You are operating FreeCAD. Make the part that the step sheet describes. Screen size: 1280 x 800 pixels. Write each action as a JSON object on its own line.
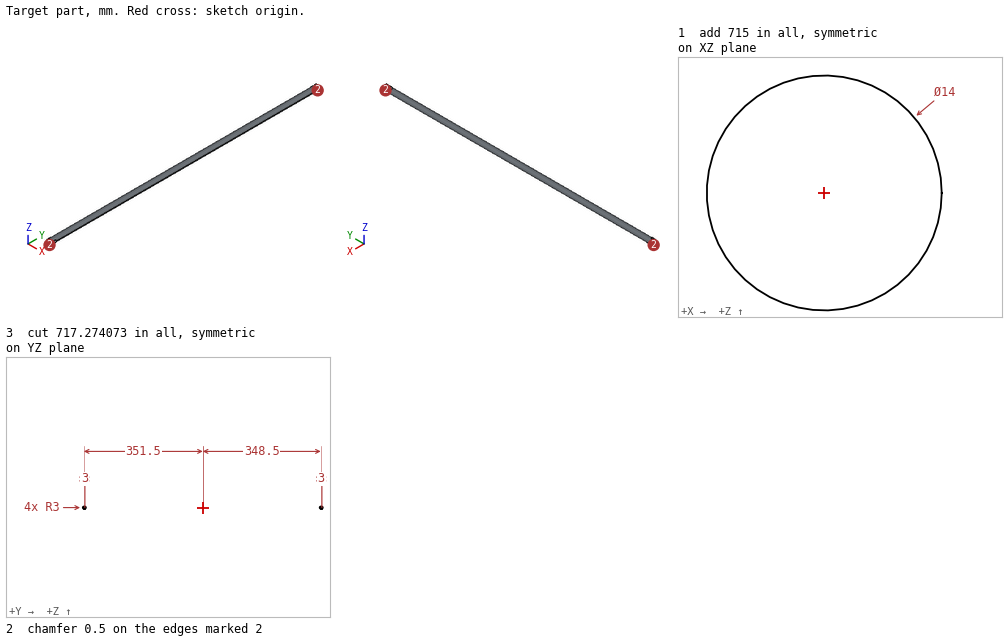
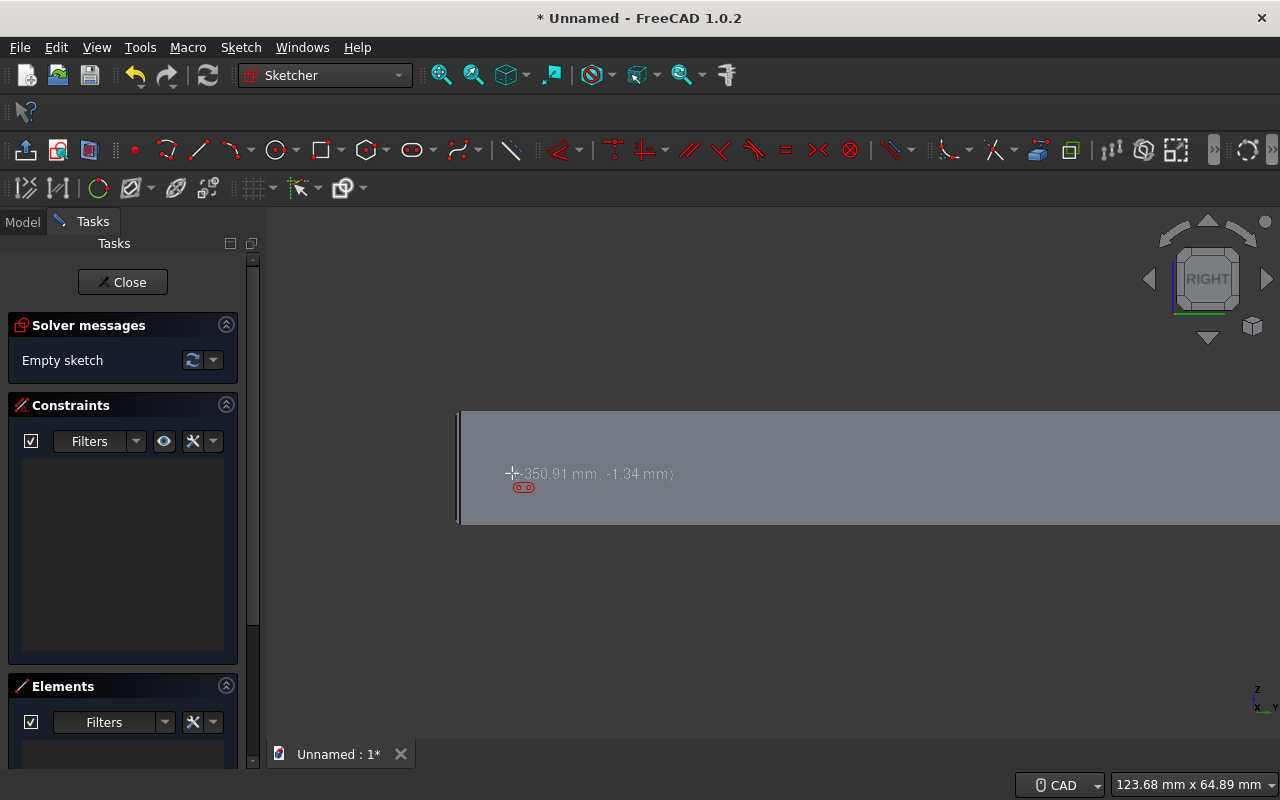
{"action": "scroll", "coordinate": [437, 474], "scroll_direction": "down", "scroll_amount": 12}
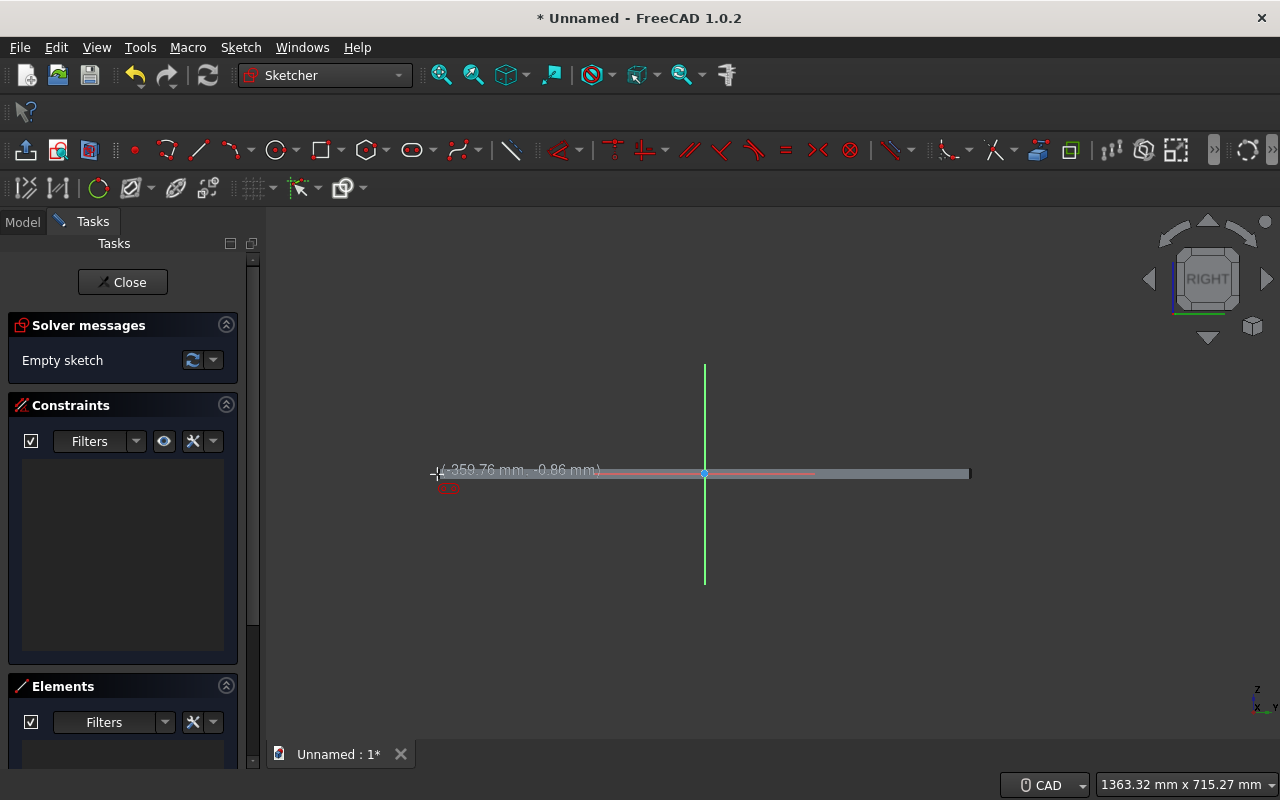
{"action": "left_click", "coordinate": [443, 474]}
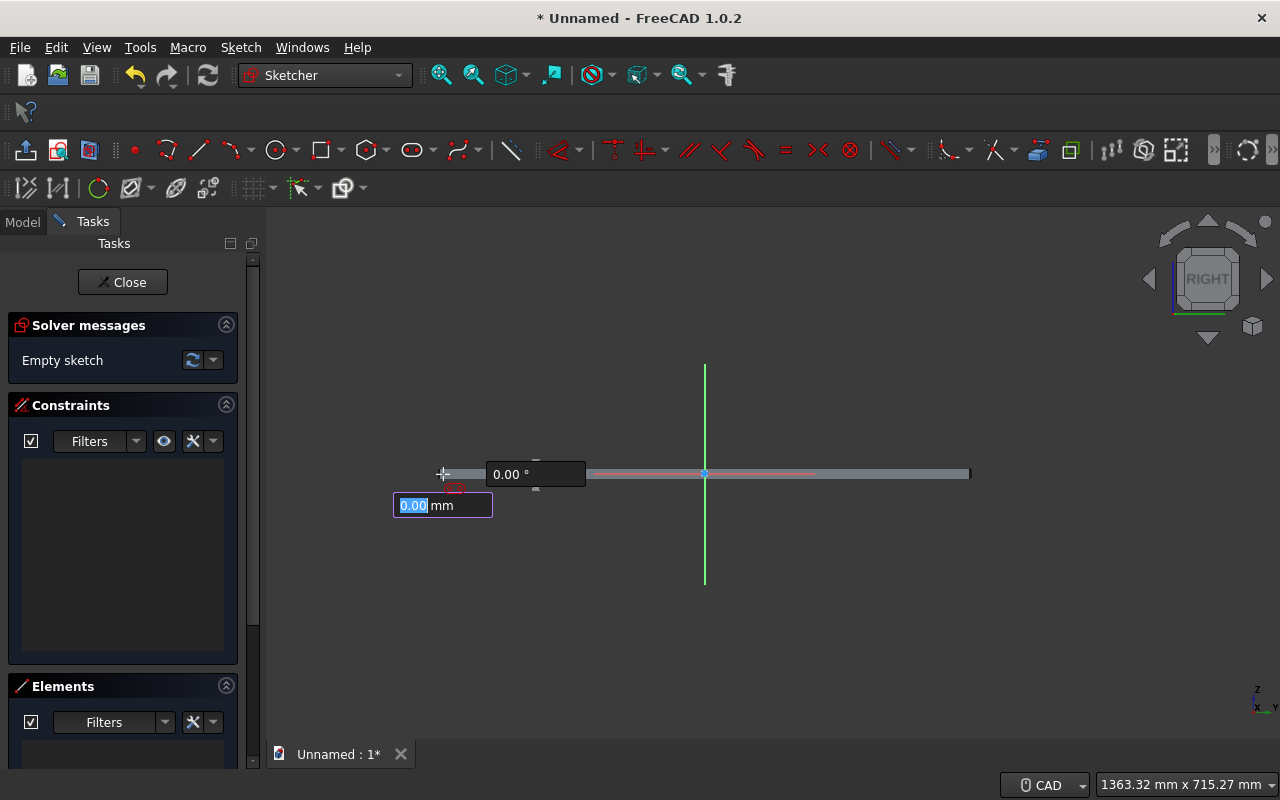
{"action": "scroll", "coordinate": [446, 474], "scroll_direction": "up", "scroll_amount": 10}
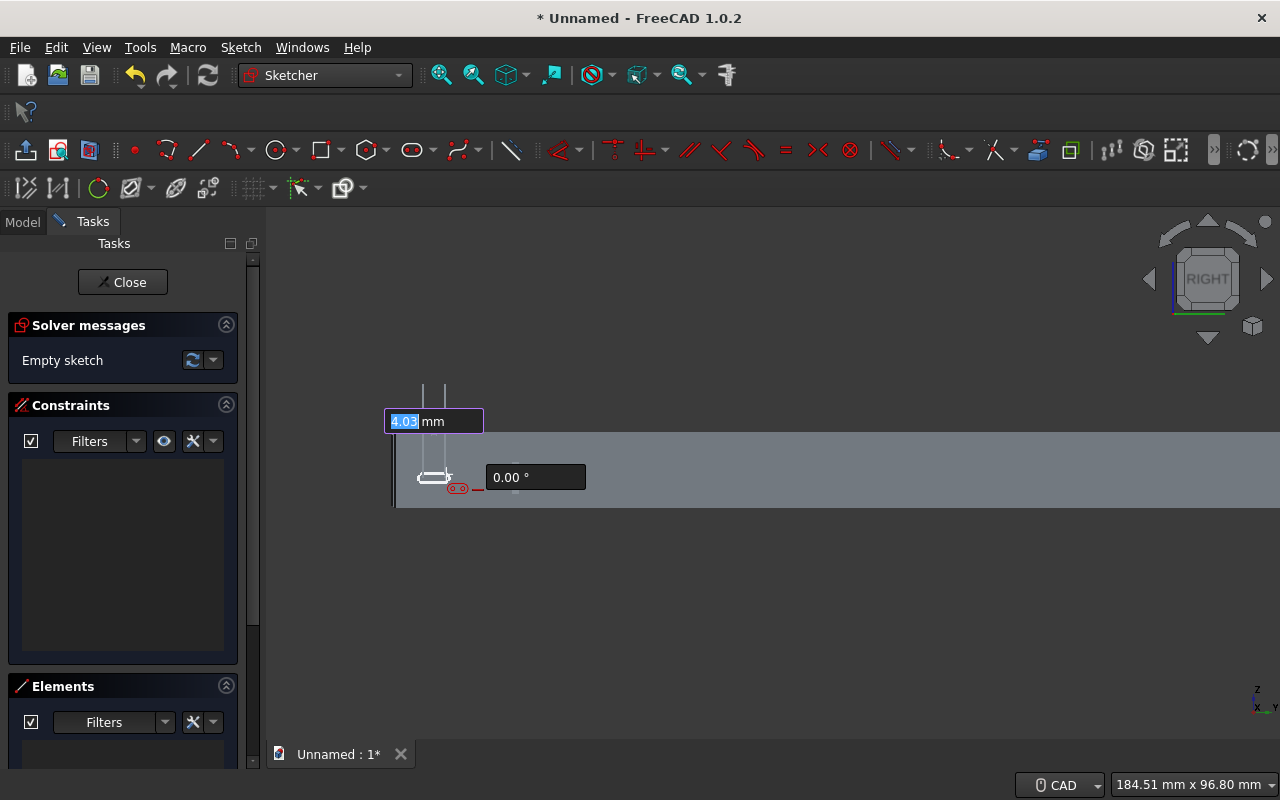
{"action": "left_click", "coordinate": [441, 461]}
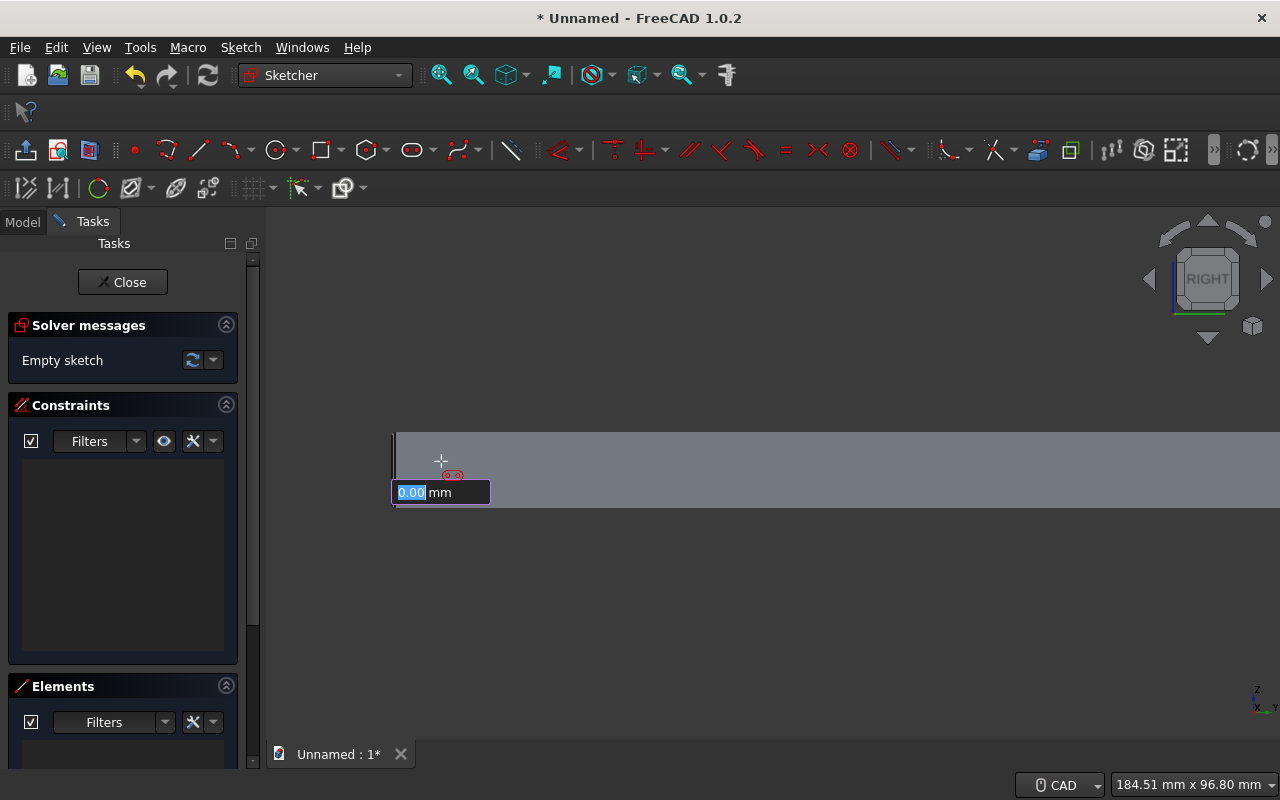
{"action": "left_click", "coordinate": [433, 454]}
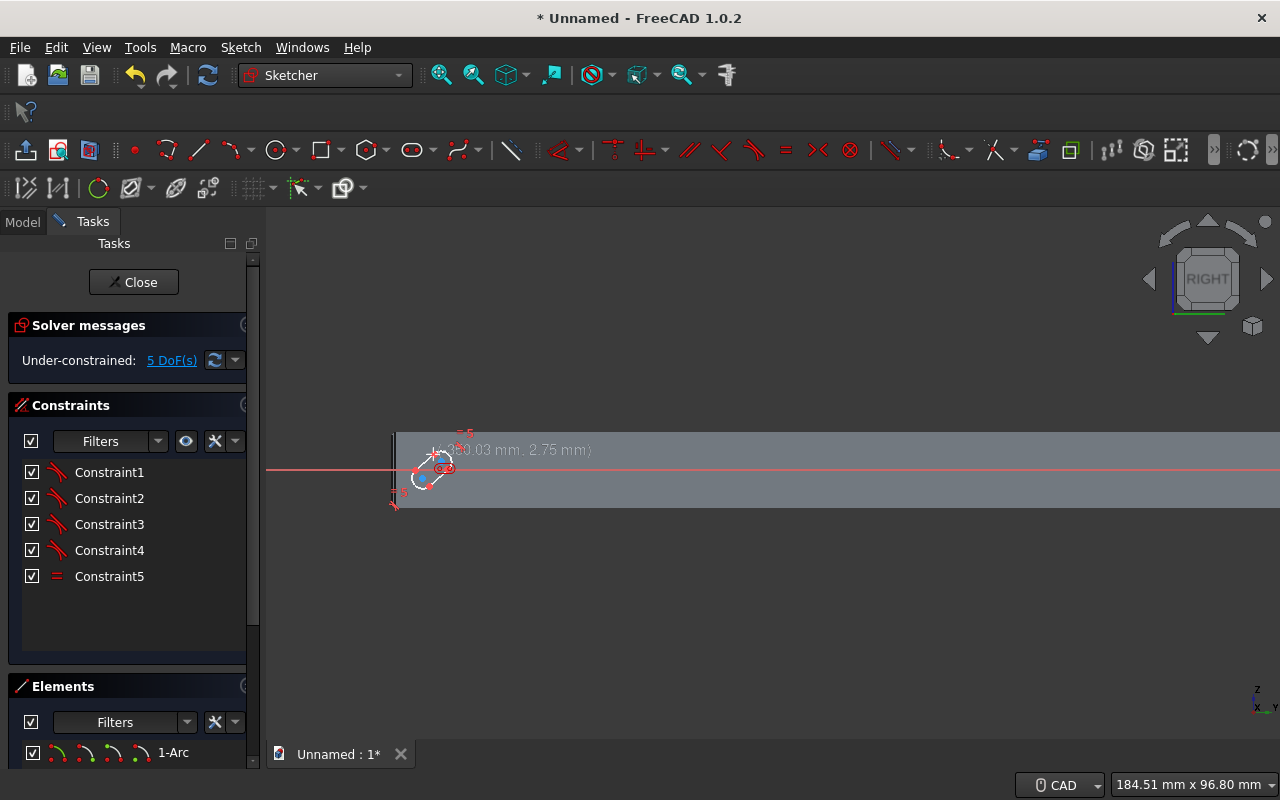
{"action": "scroll", "coordinate": [446, 473], "scroll_direction": "down", "scroll_amount": 10}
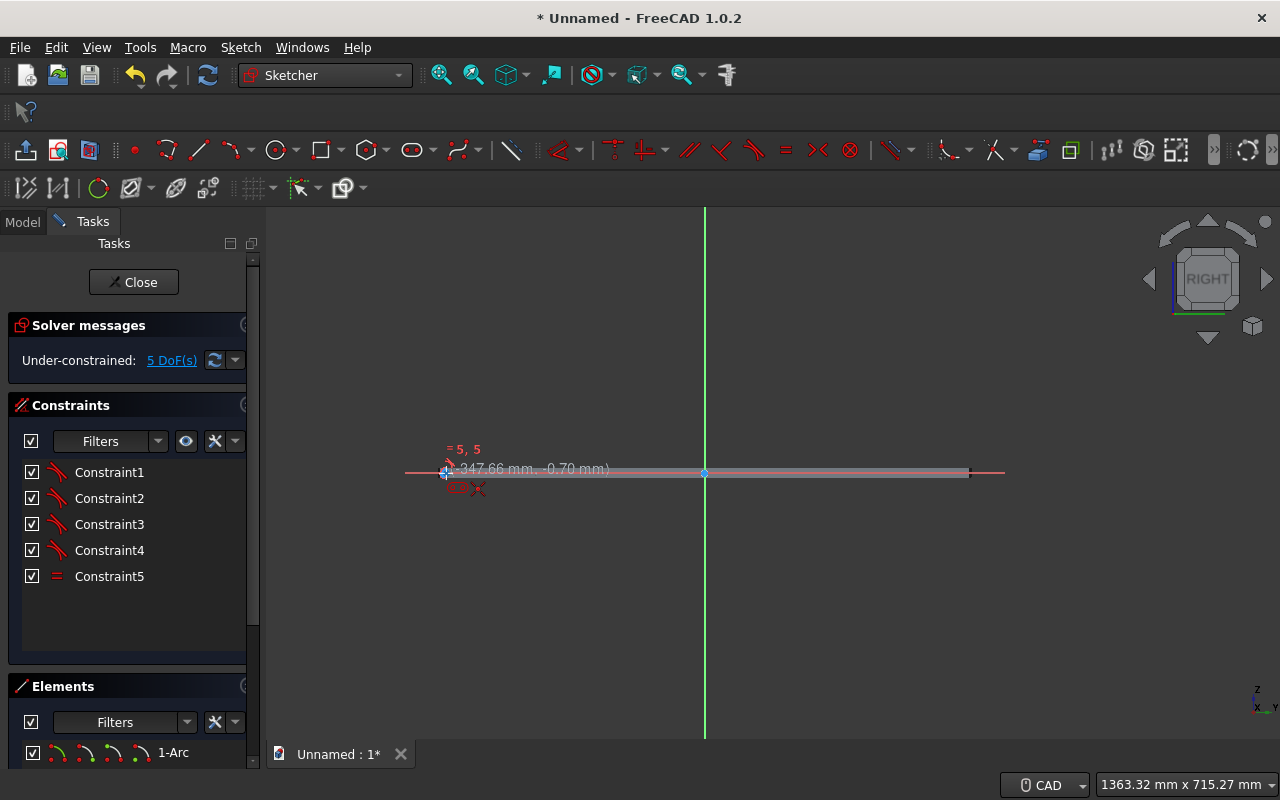
{"action": "scroll", "coordinate": [964, 473], "scroll_direction": "up", "scroll_amount": 12}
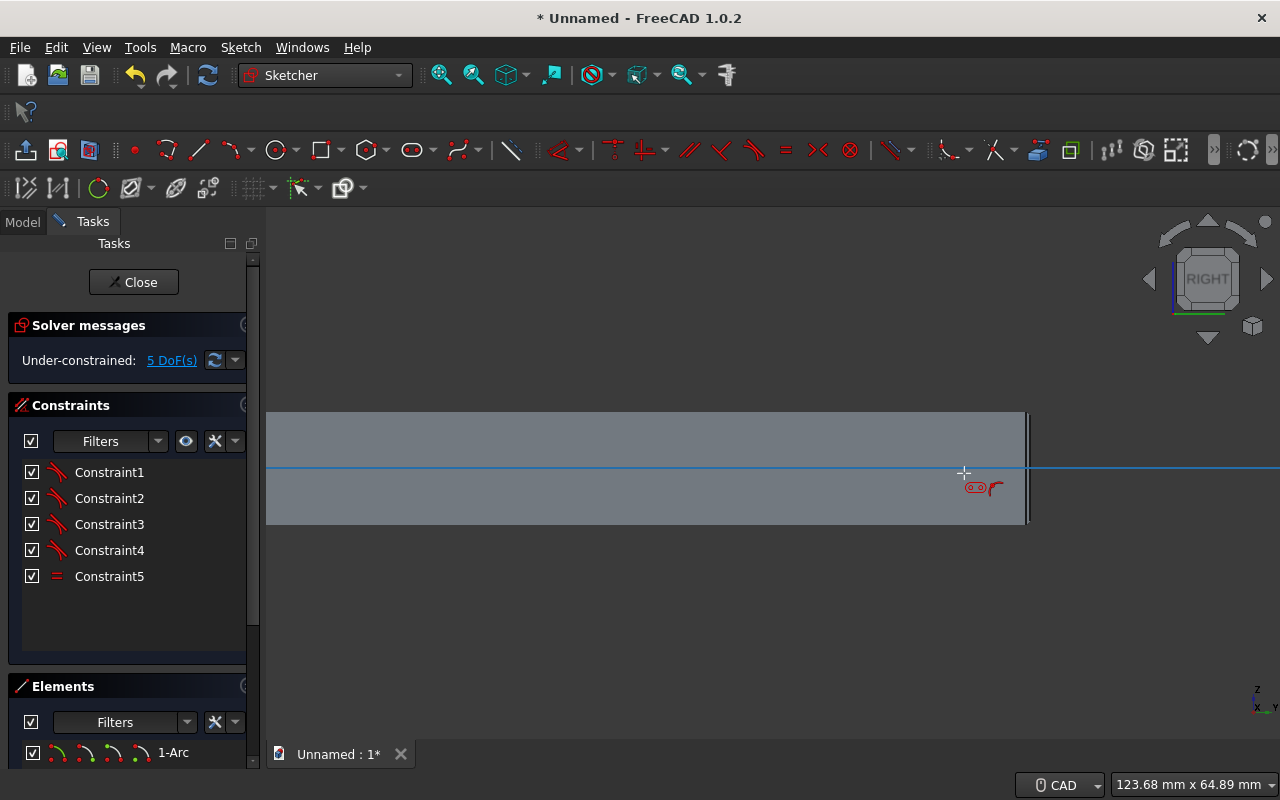
{"action": "scroll", "coordinate": [964, 473], "scroll_direction": "down", "scroll_amount": 12}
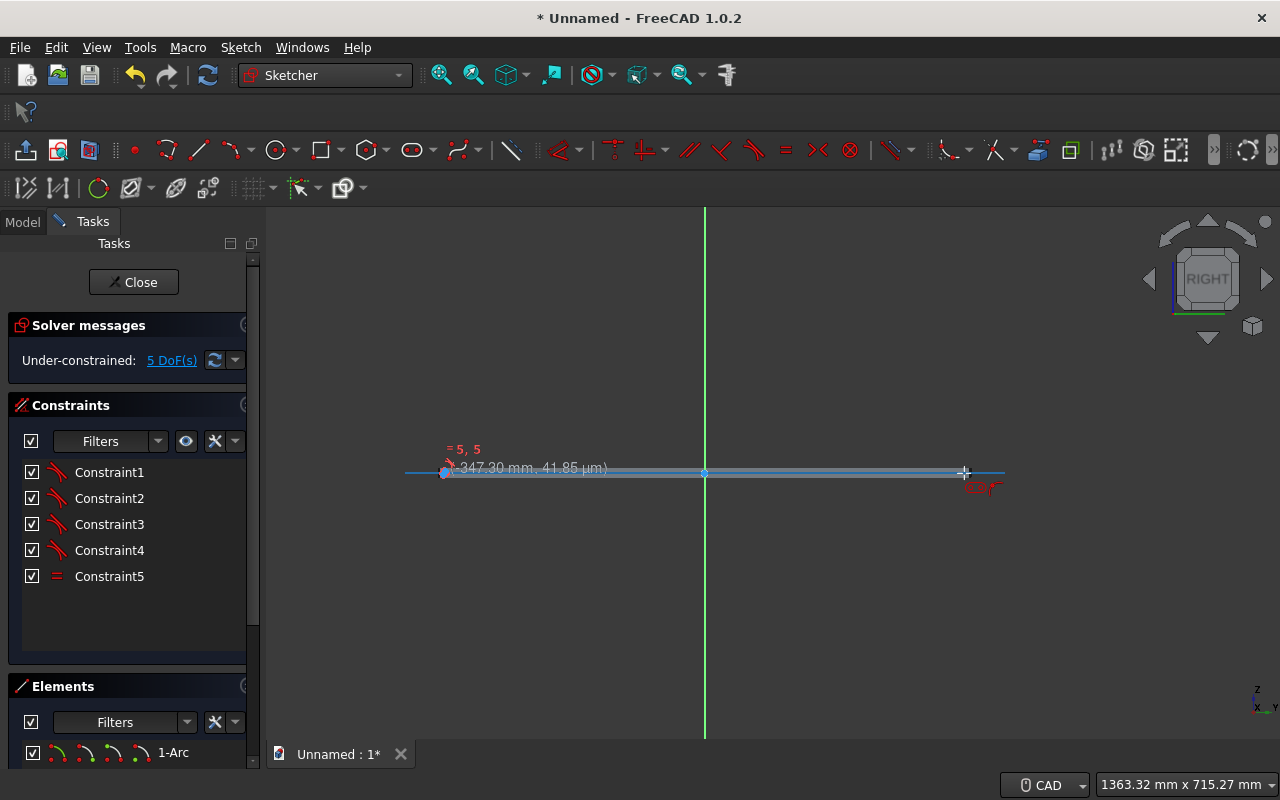
{"action": "left_click", "coordinate": [964, 473]}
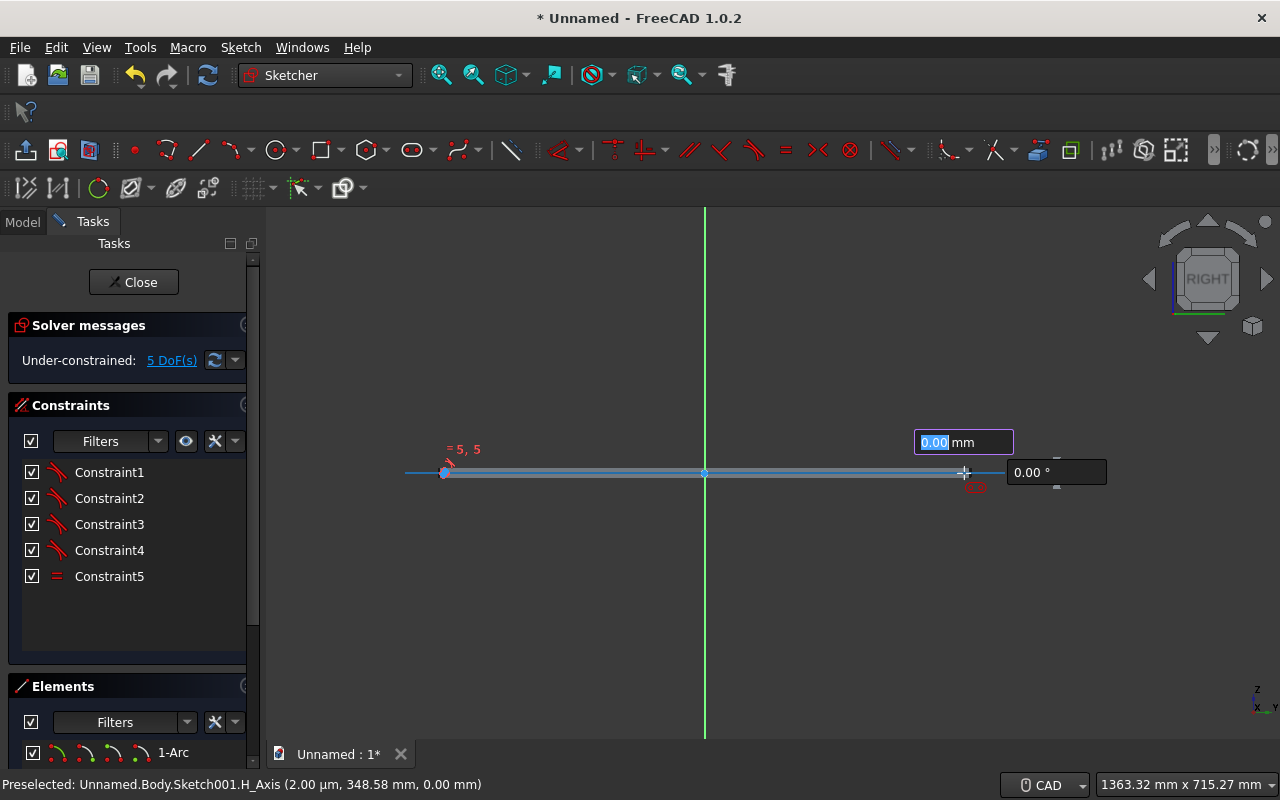
{"action": "scroll", "coordinate": [966, 473], "scroll_direction": "up", "scroll_amount": 10}